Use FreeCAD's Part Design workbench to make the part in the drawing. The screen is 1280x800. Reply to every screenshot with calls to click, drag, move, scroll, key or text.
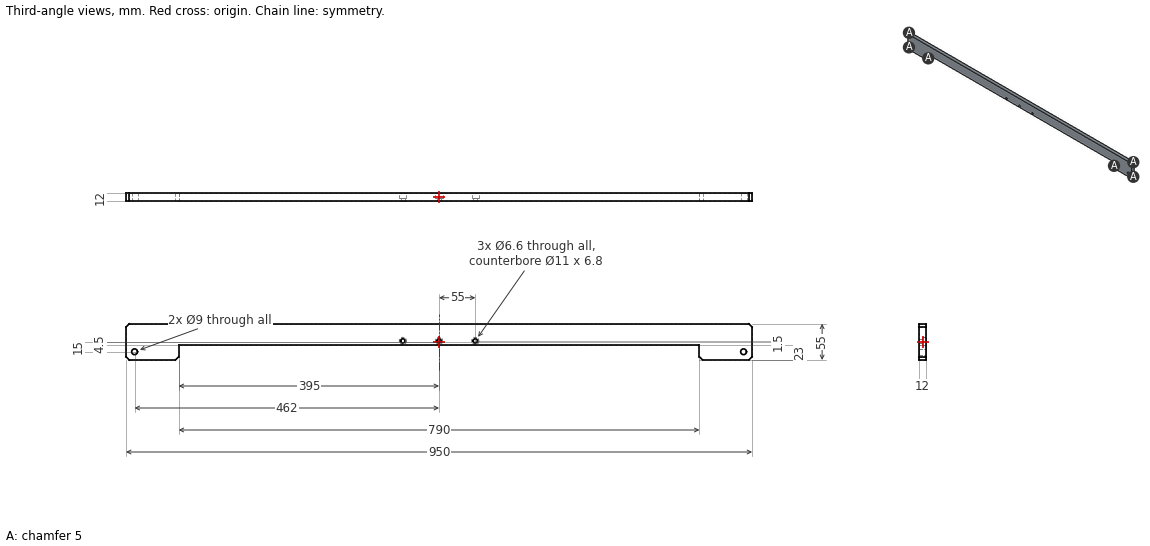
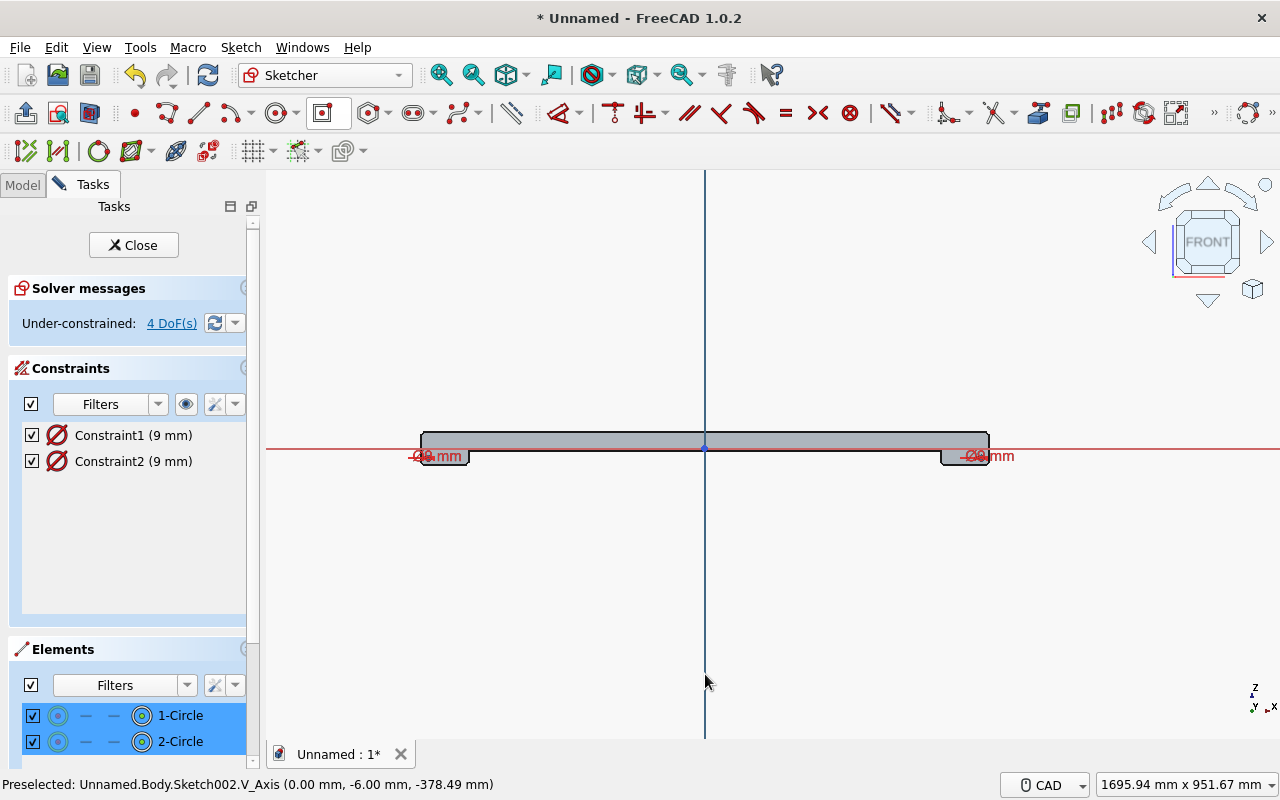
key(s)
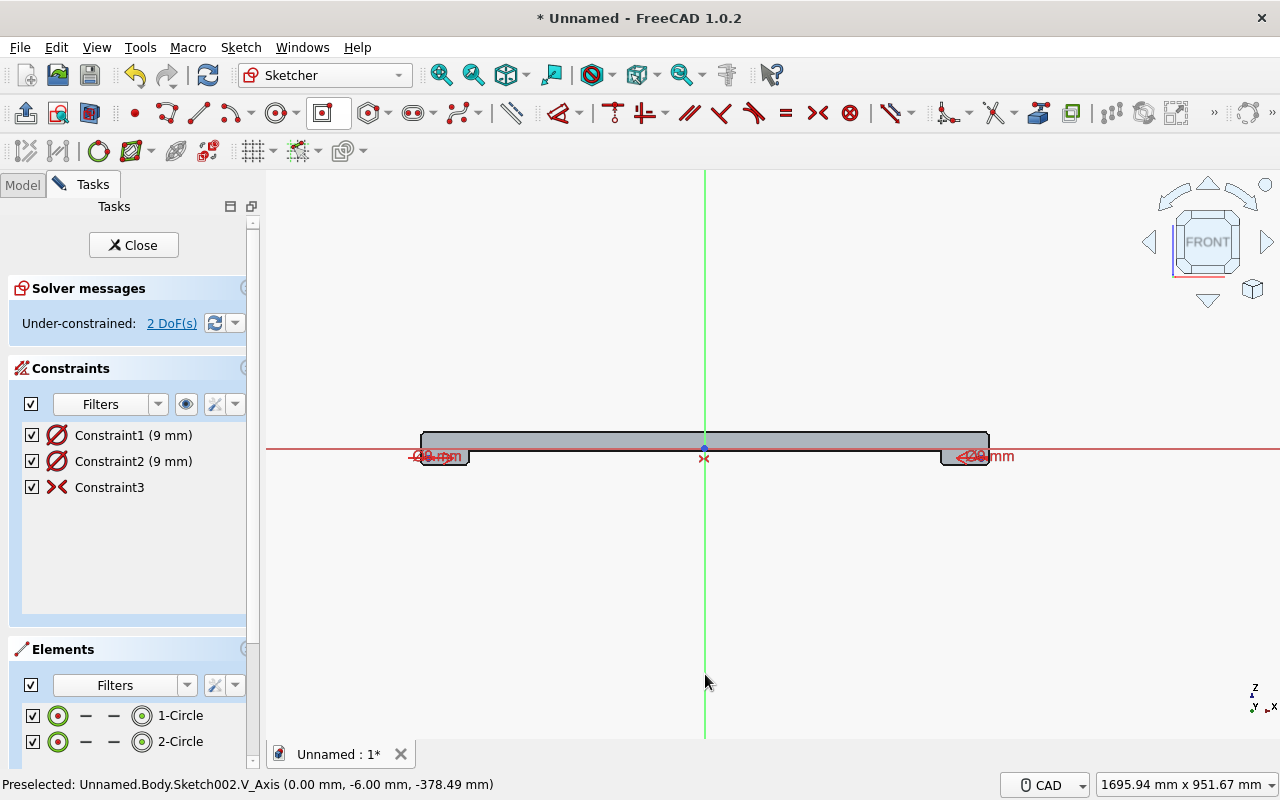
key(d)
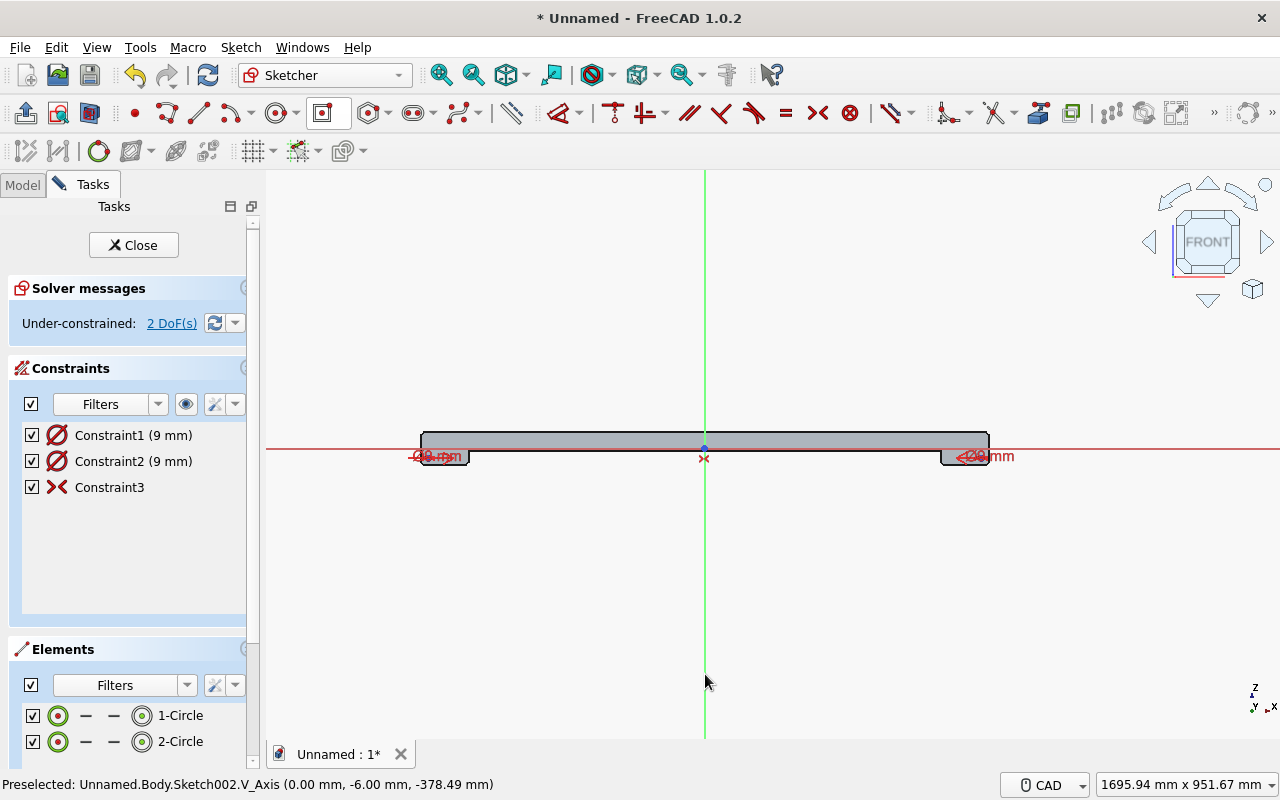
scroll(428, 458, up, 8)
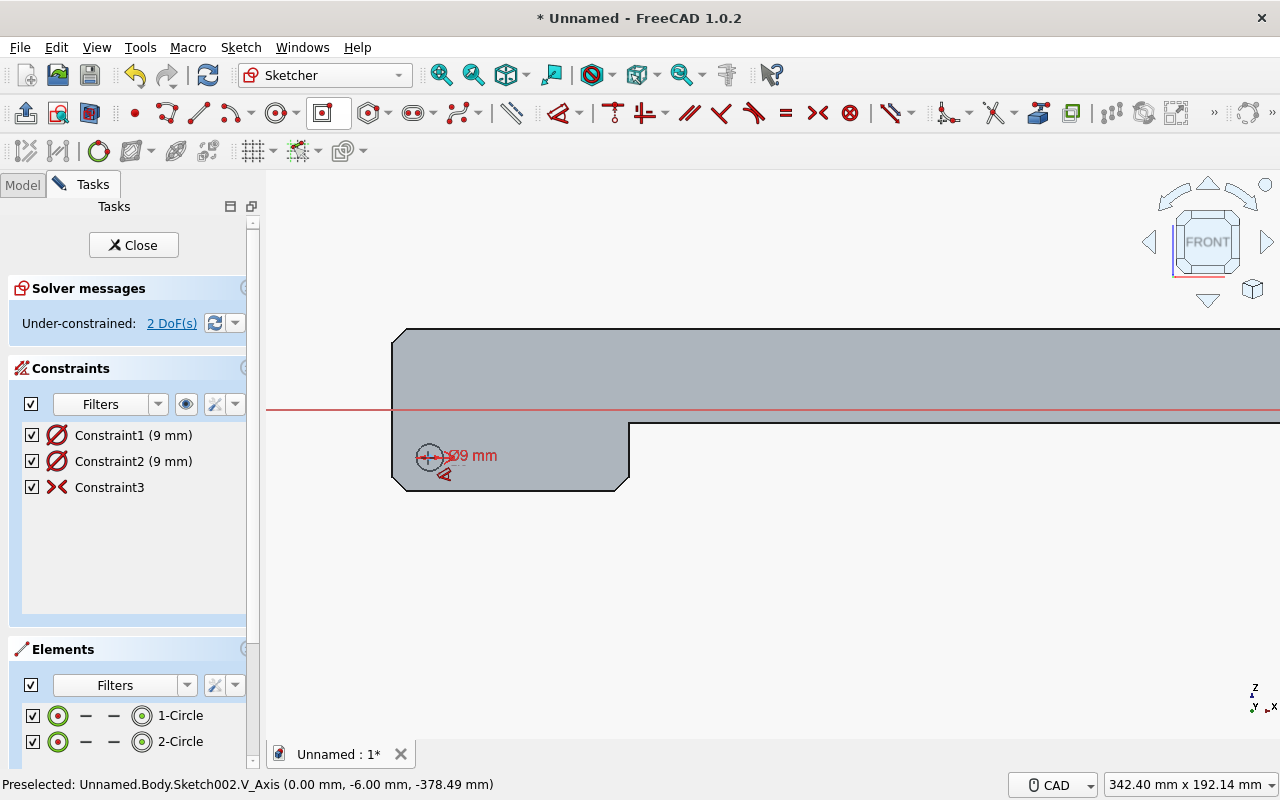
click(430, 458)
click(396, 434)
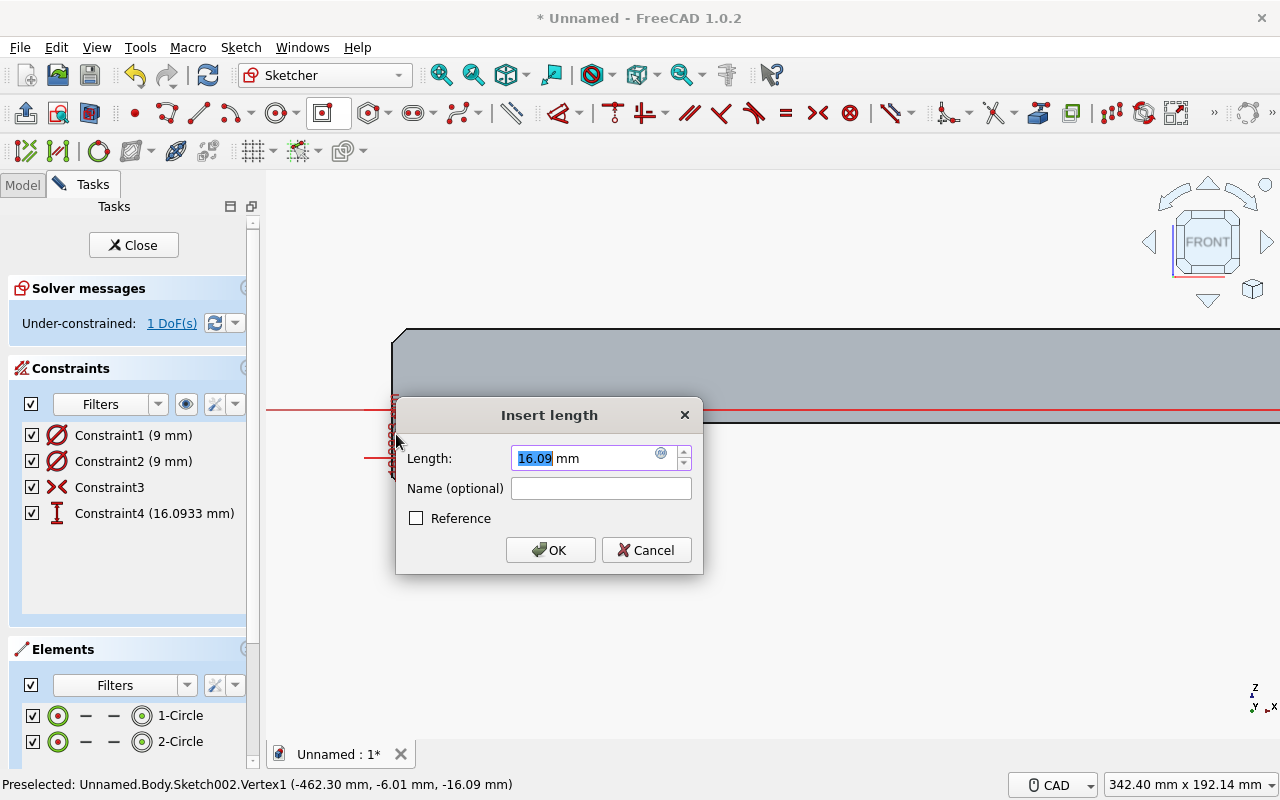
text(15)
key(Return)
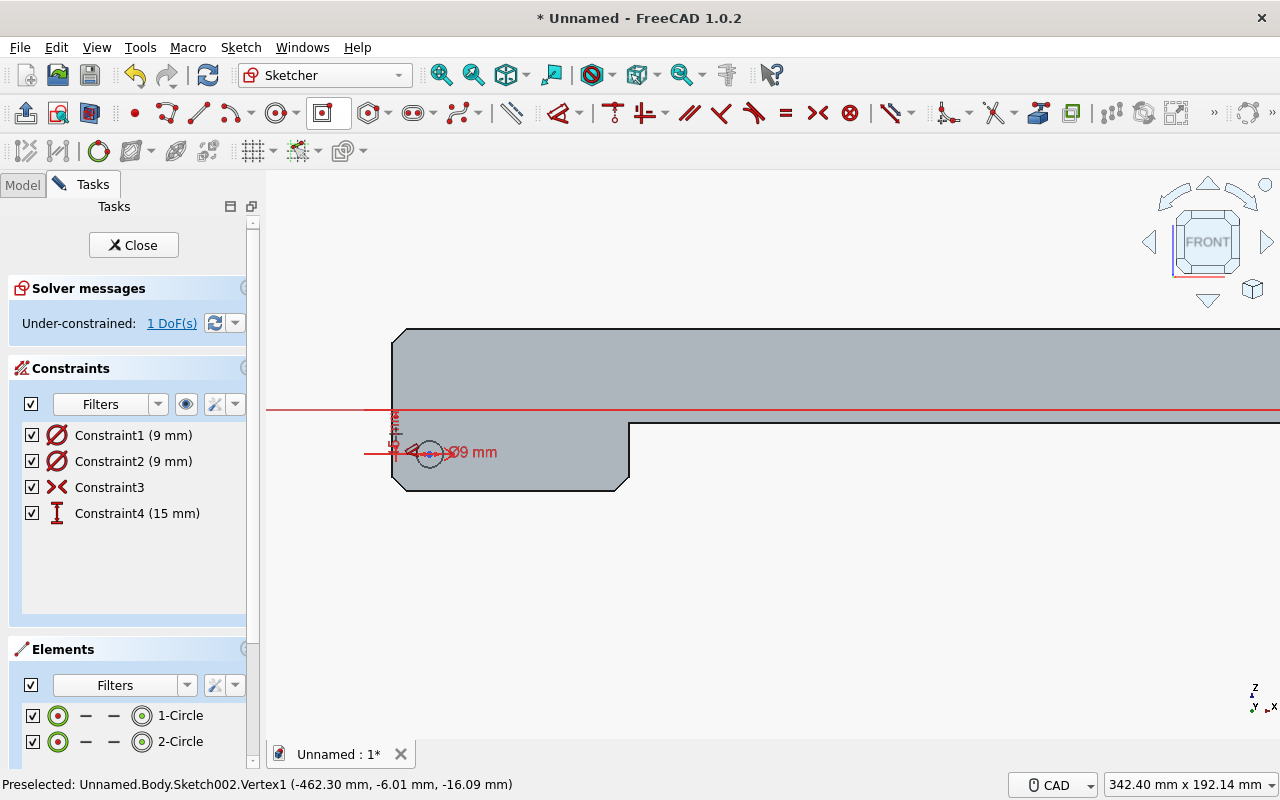
scroll(428, 458, down, 8)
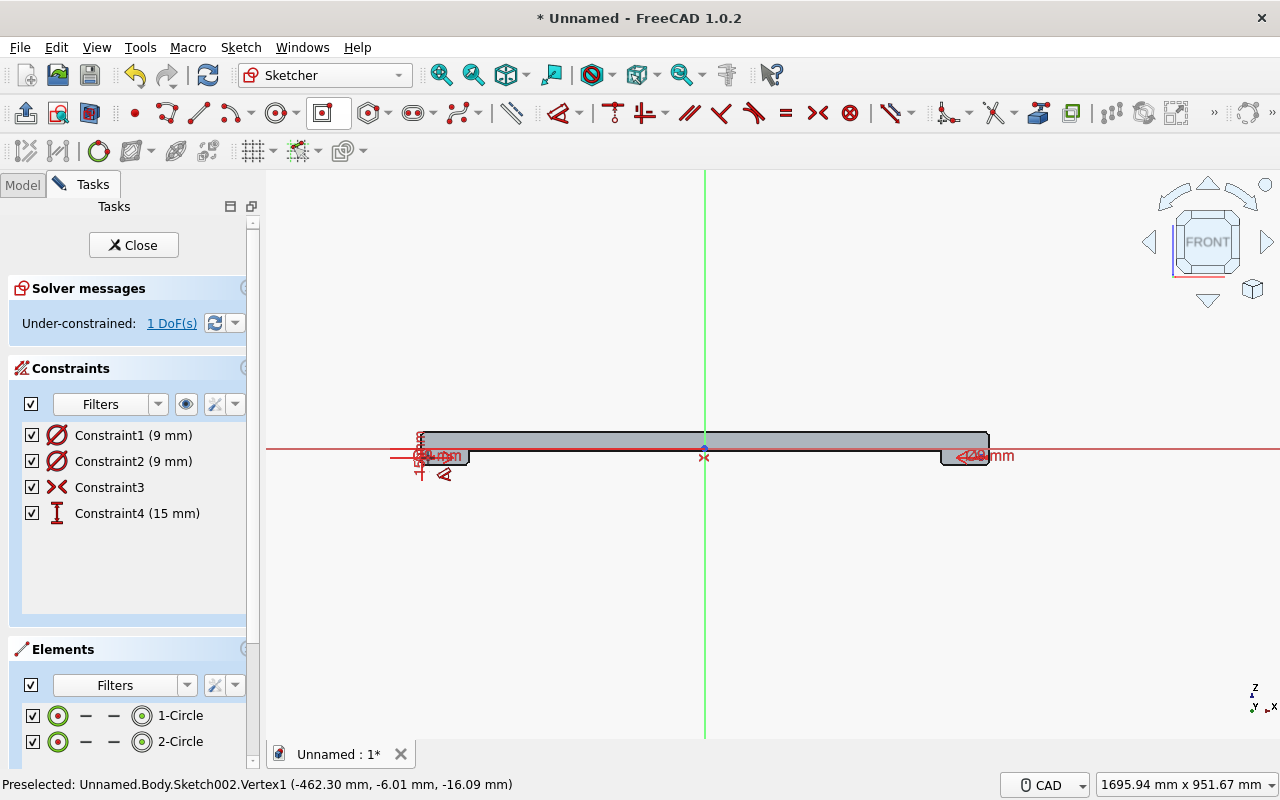
click(428, 458)
click(567, 415)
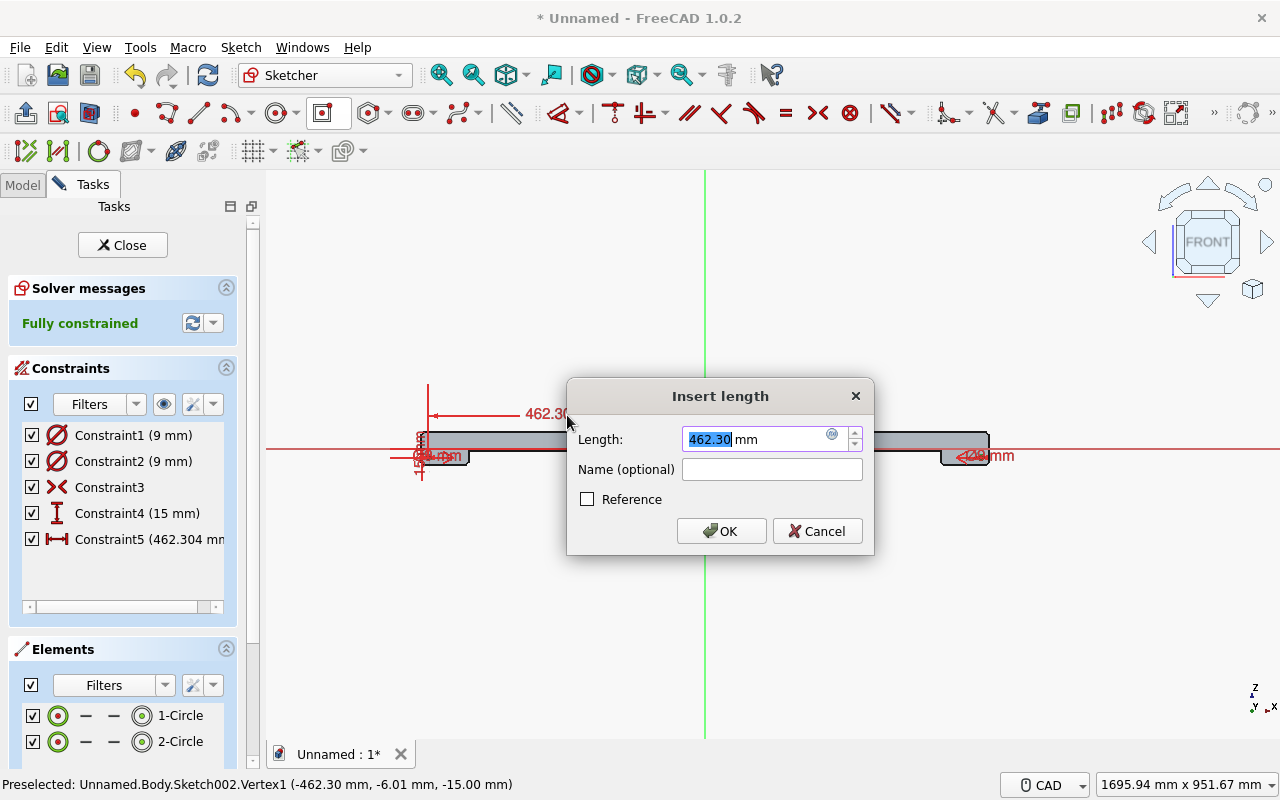
text(462)
key(Return)
key(Escape)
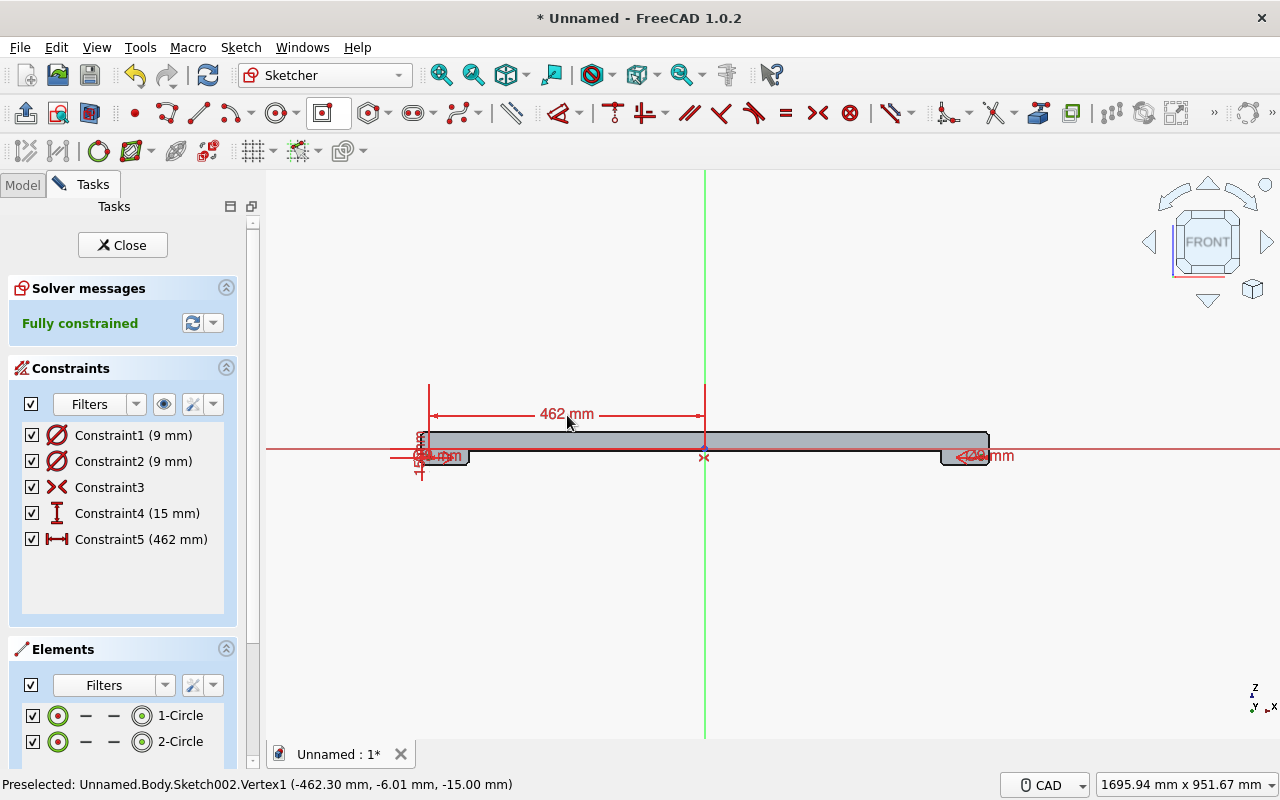
click(123, 245)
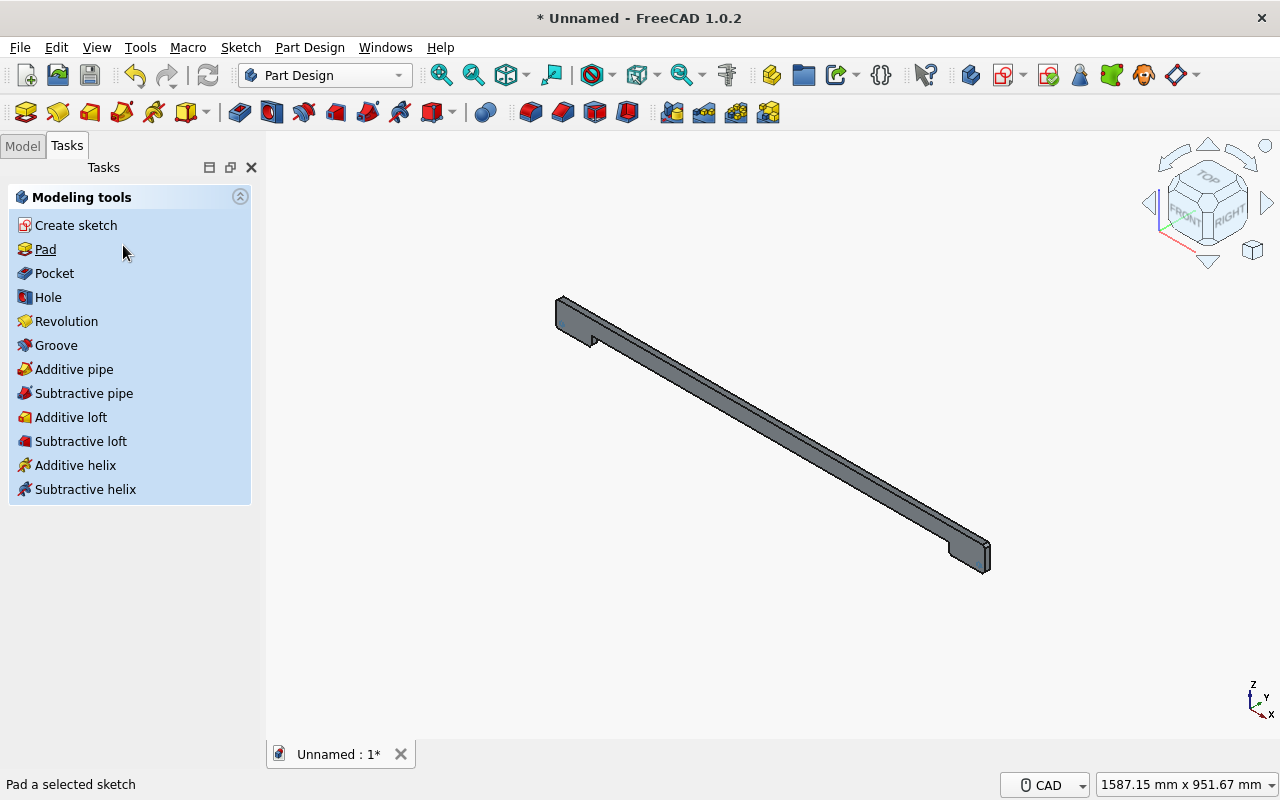
click(272, 112)